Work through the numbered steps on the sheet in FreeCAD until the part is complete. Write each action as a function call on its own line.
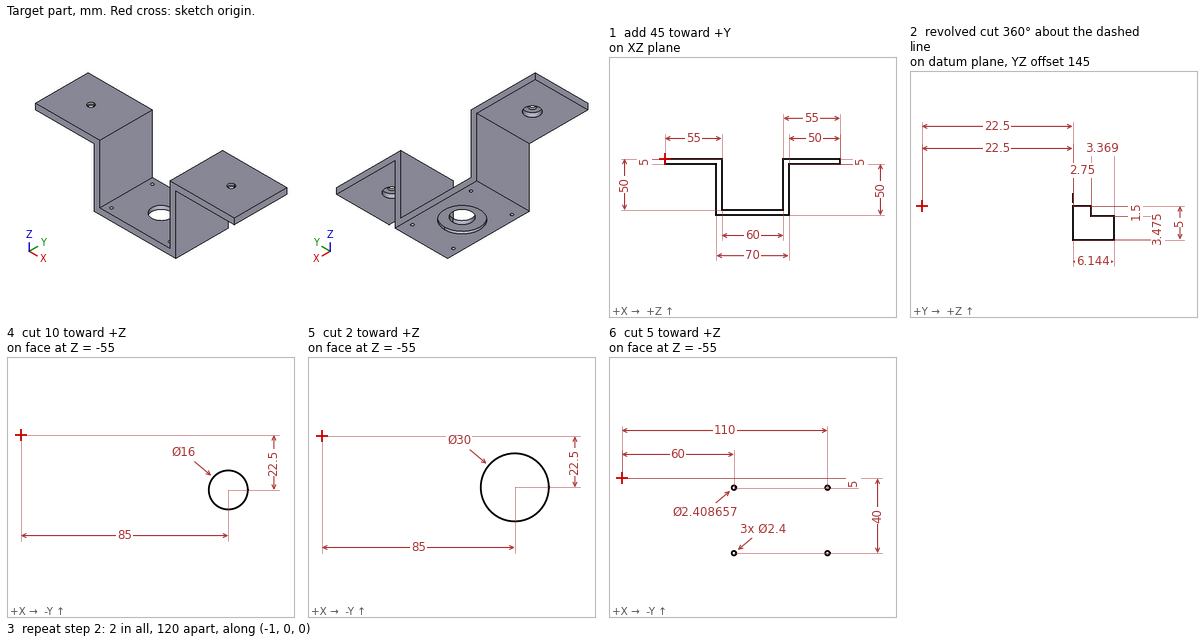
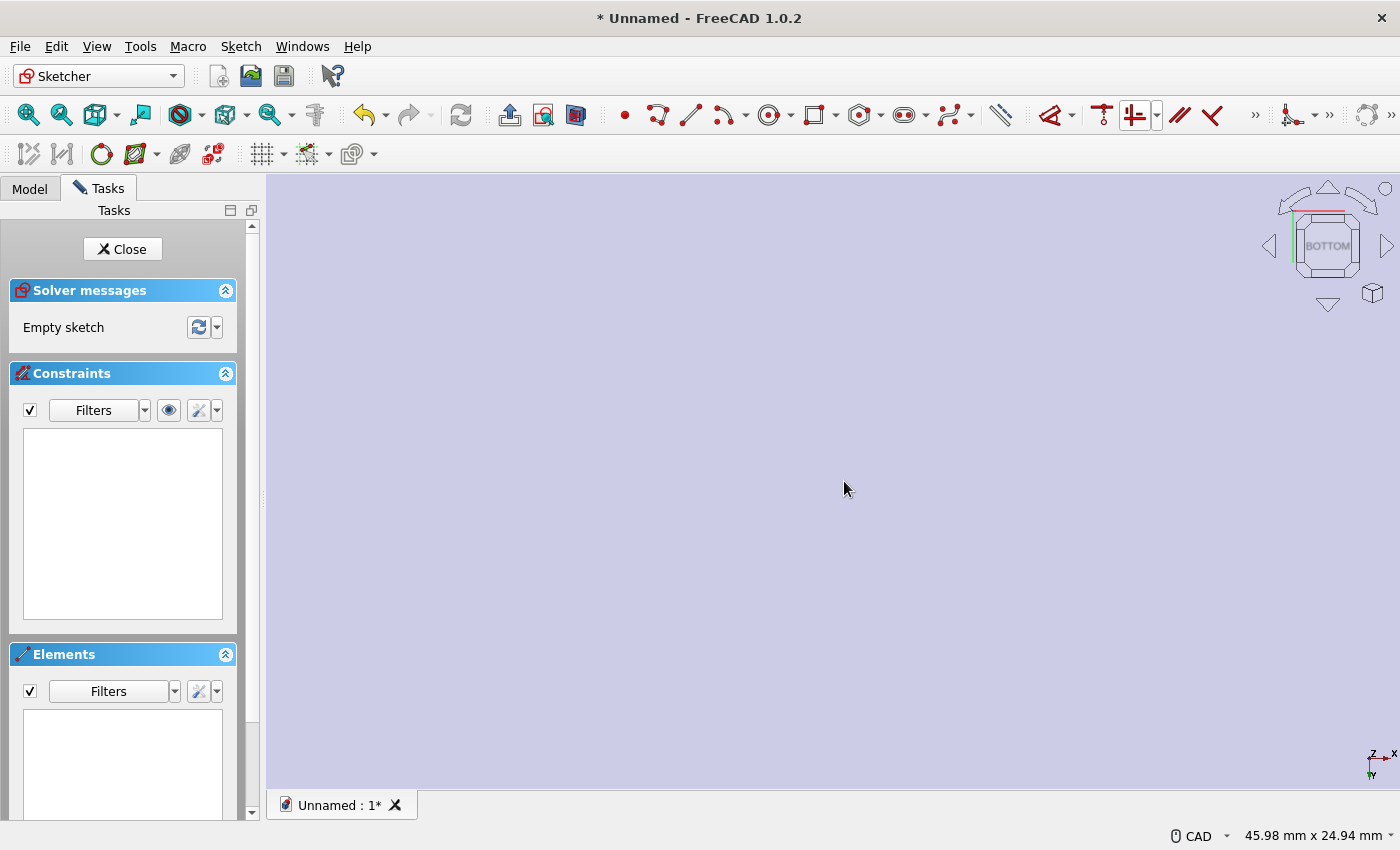
click(768, 116)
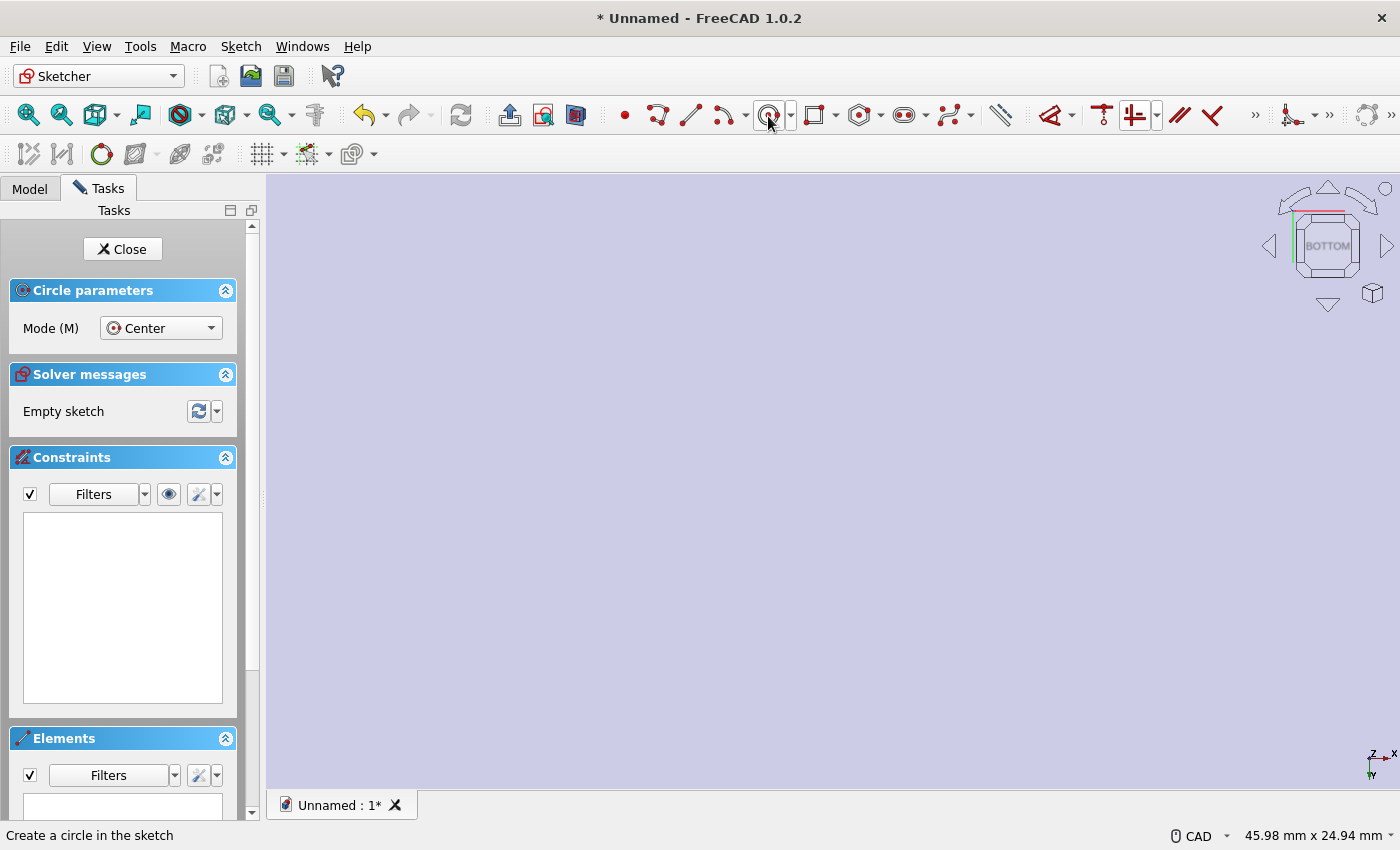
click(759, 481)
click(899, 342)
key(Escape)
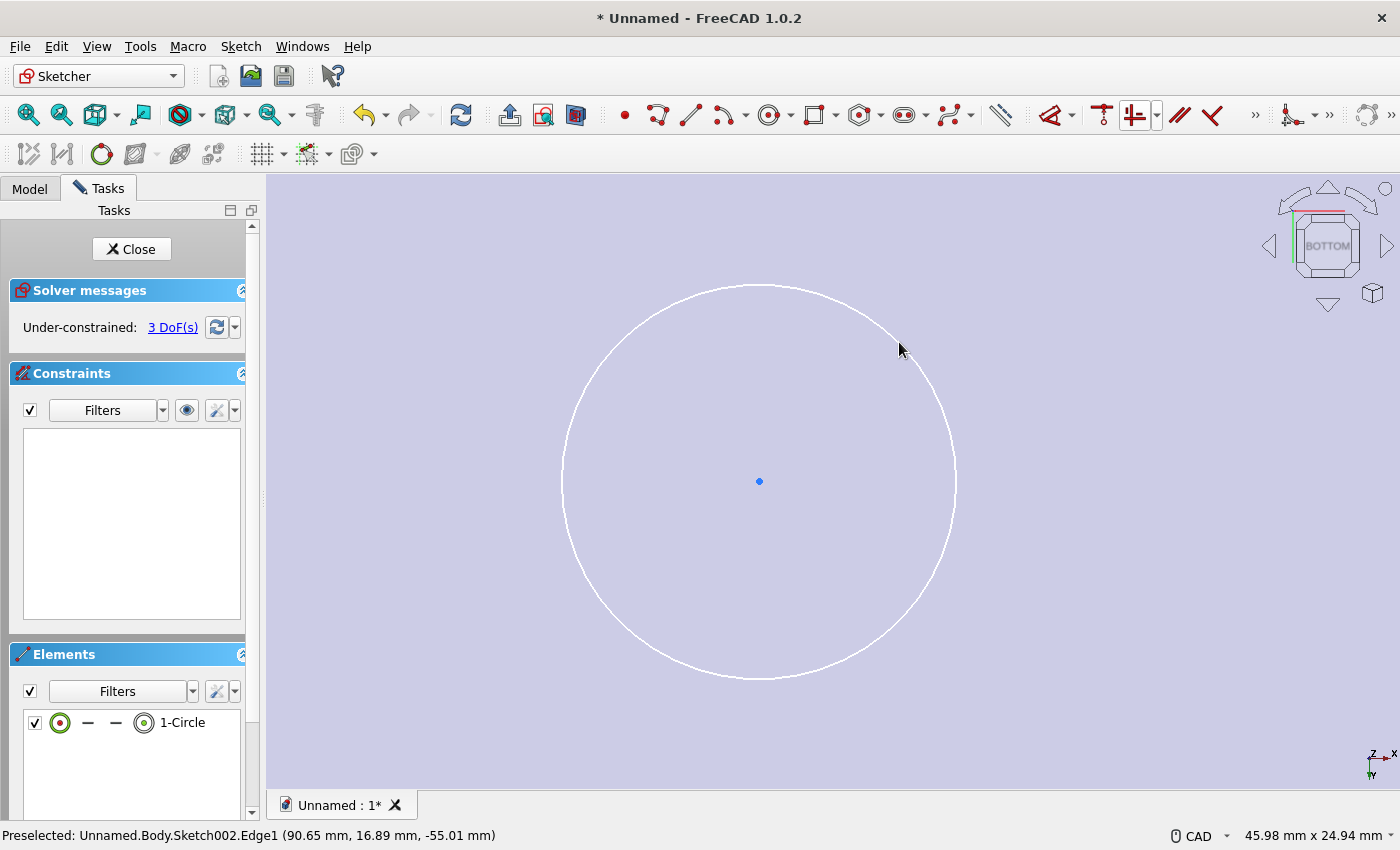
key(d)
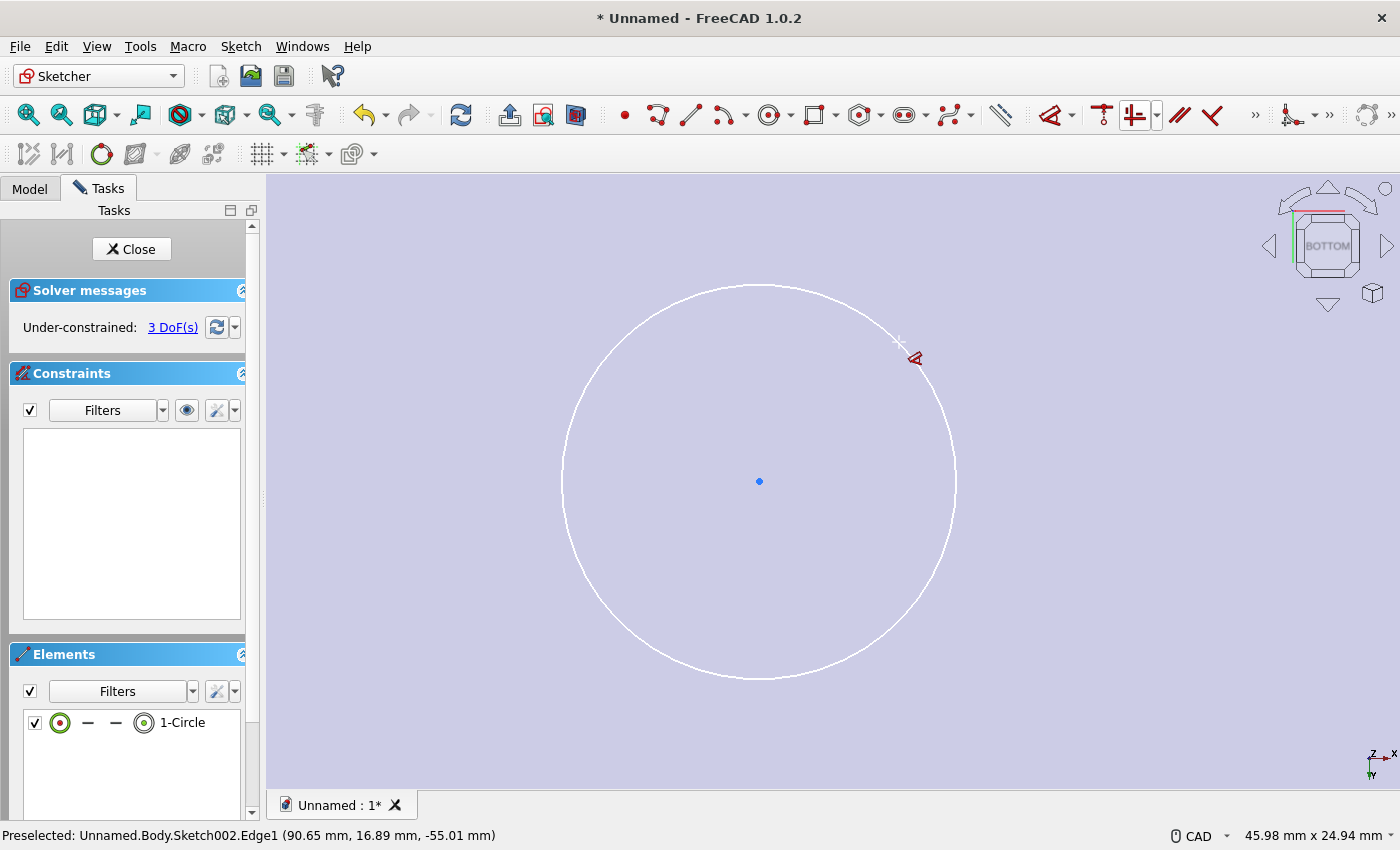
click(898, 342)
click(921, 319)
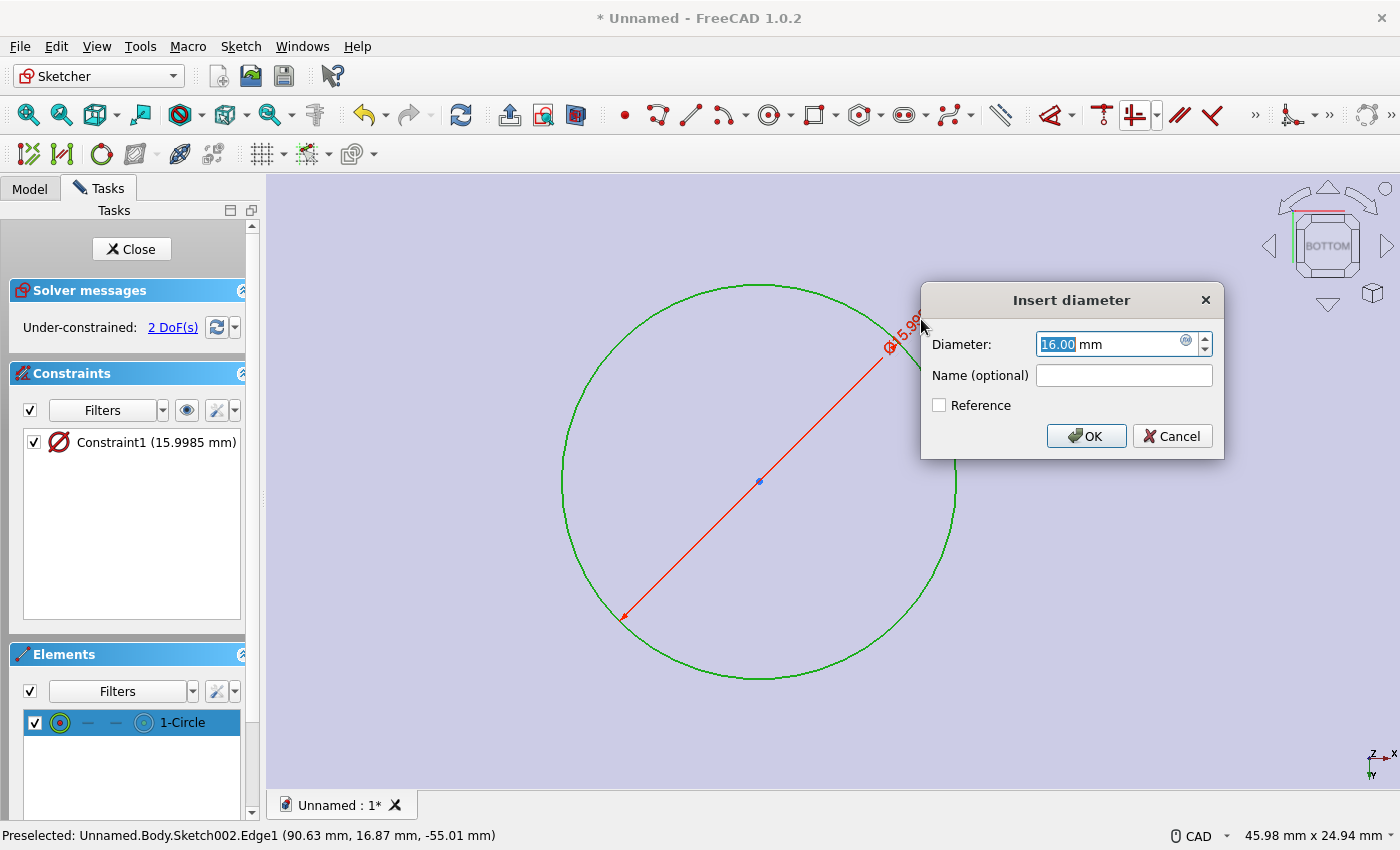
text(16)
key(Return)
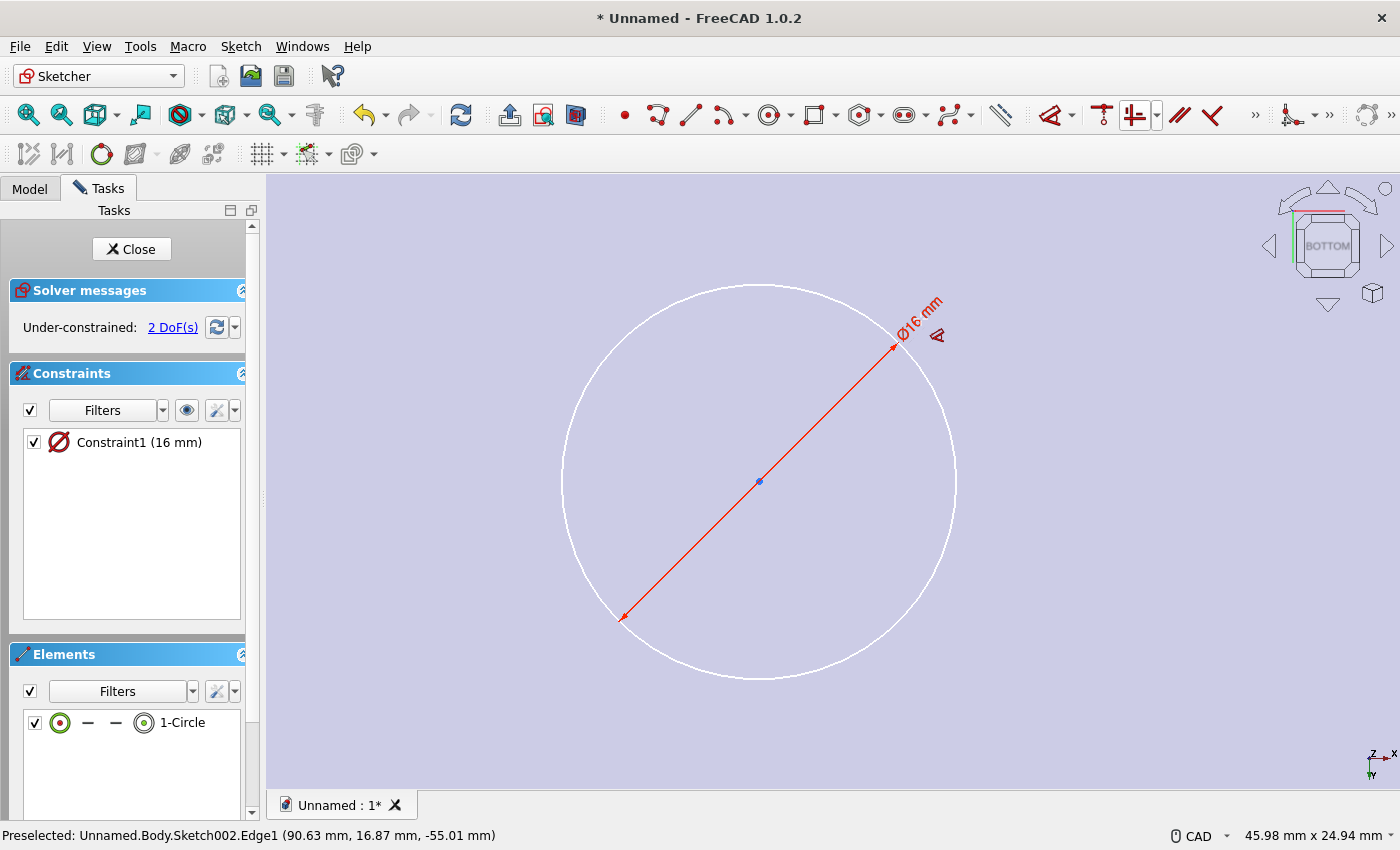
click(759, 482)
click(527, 516)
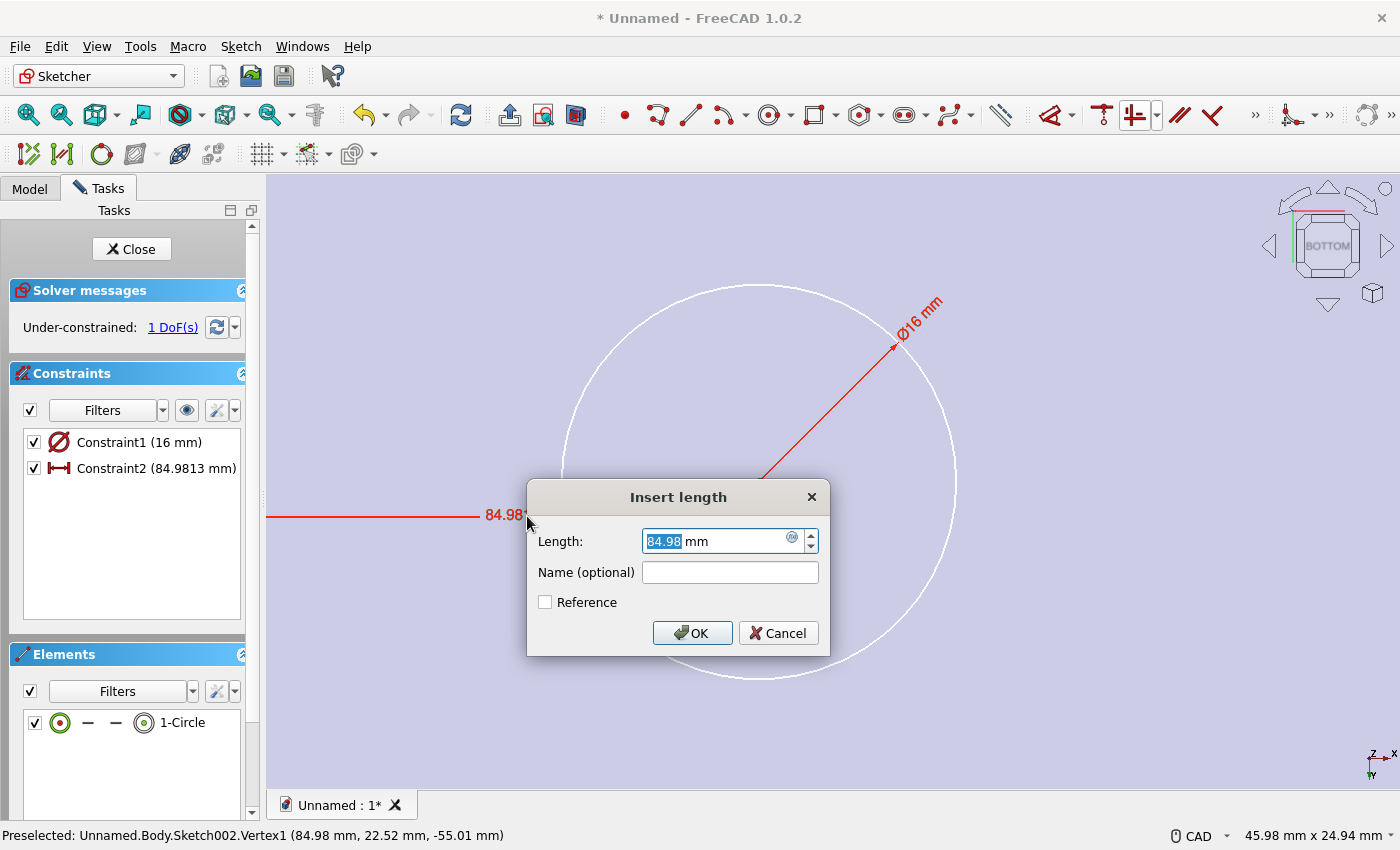
text(85)
key(Return)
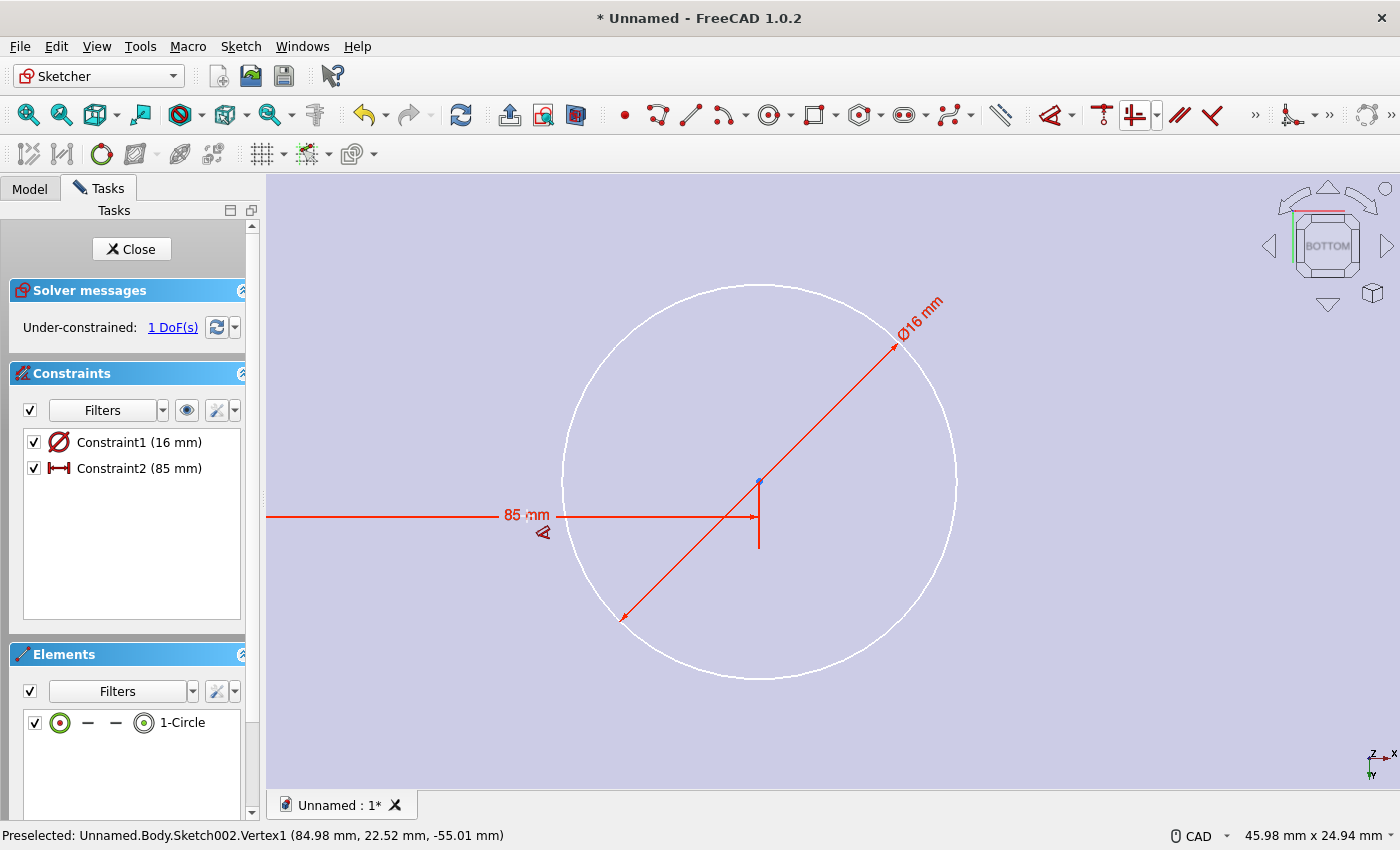
click(759, 482)
click(793, 342)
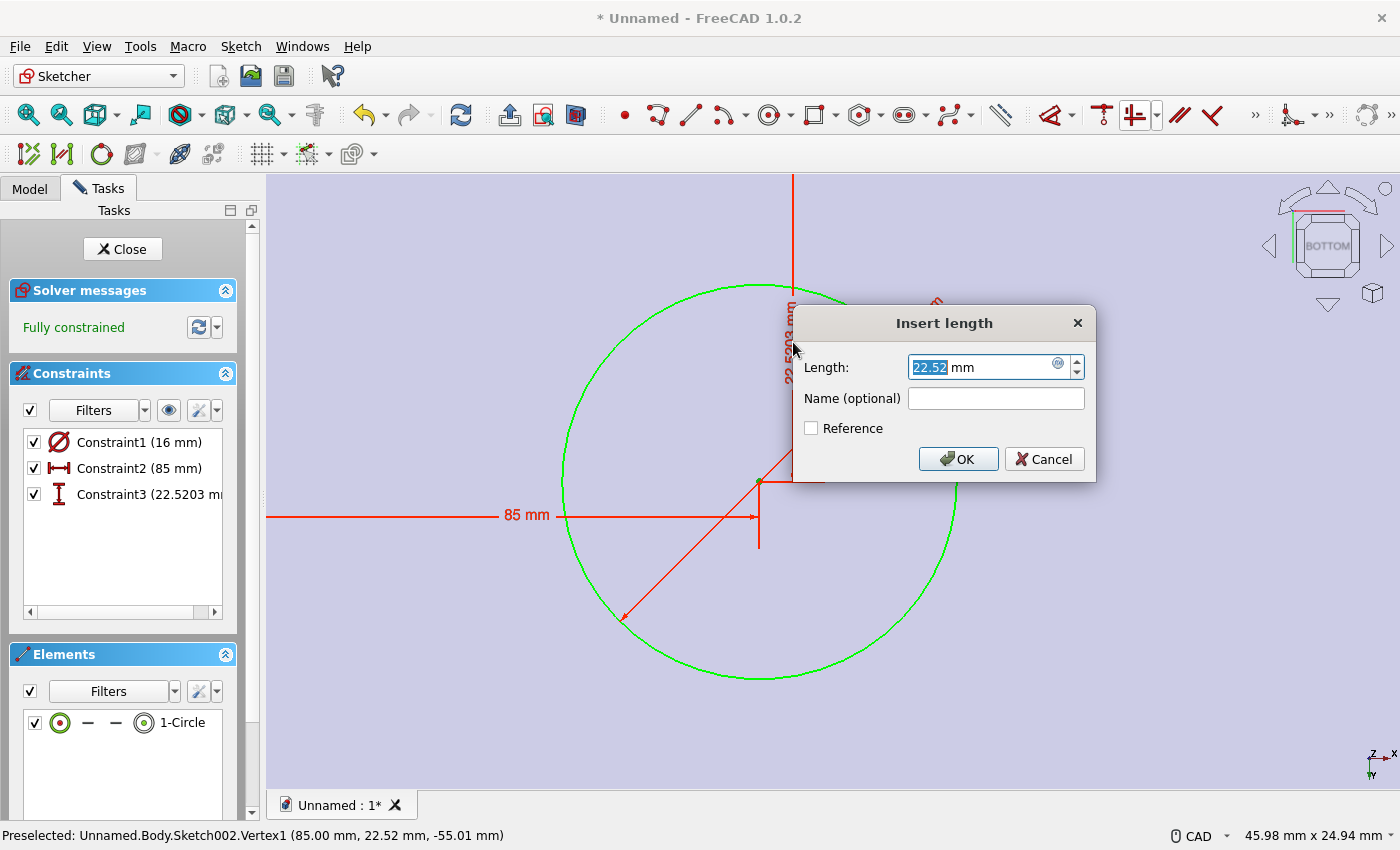
text(22.5)
key(Return)
key(Escape)